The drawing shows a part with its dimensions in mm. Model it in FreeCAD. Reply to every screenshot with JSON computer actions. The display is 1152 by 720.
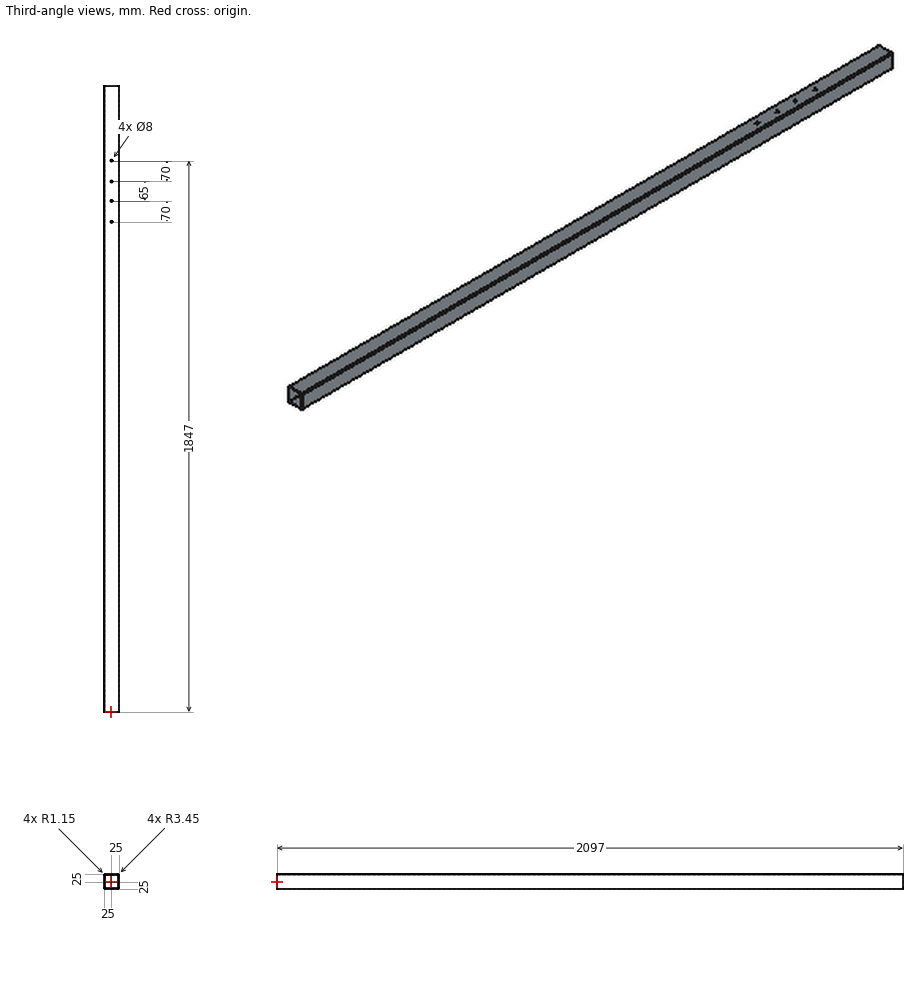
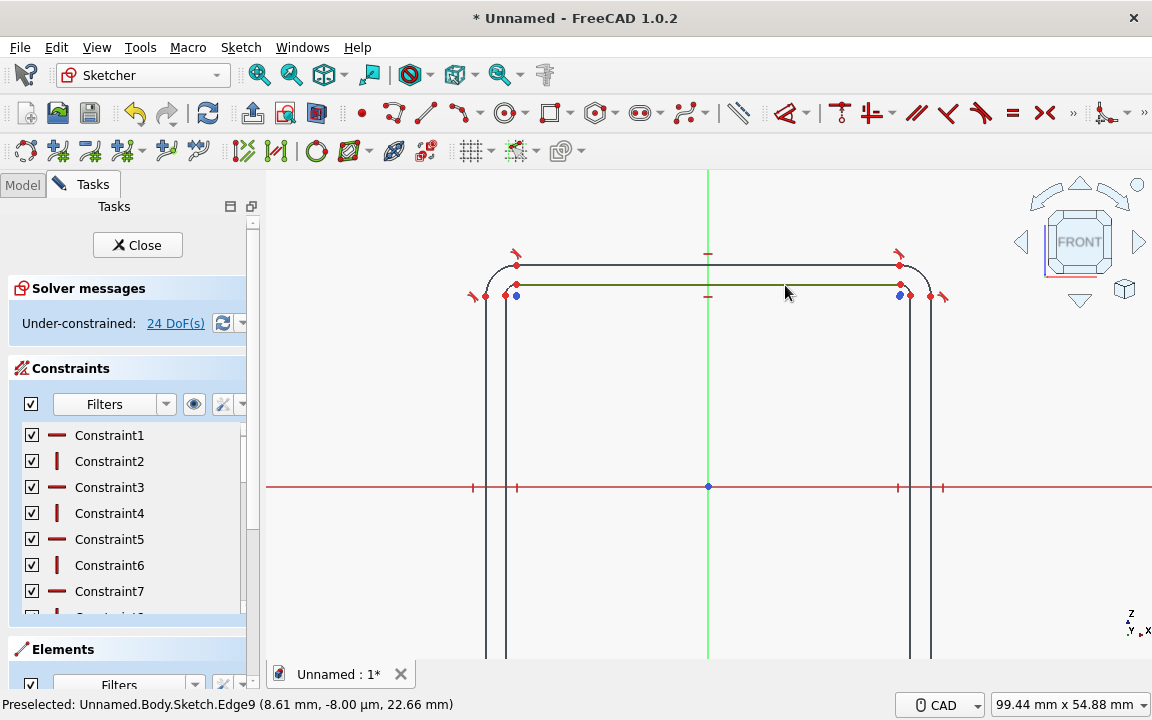
{"action": "scroll", "coordinate": [509, 288], "scroll_direction": "up", "scroll_amount": 3}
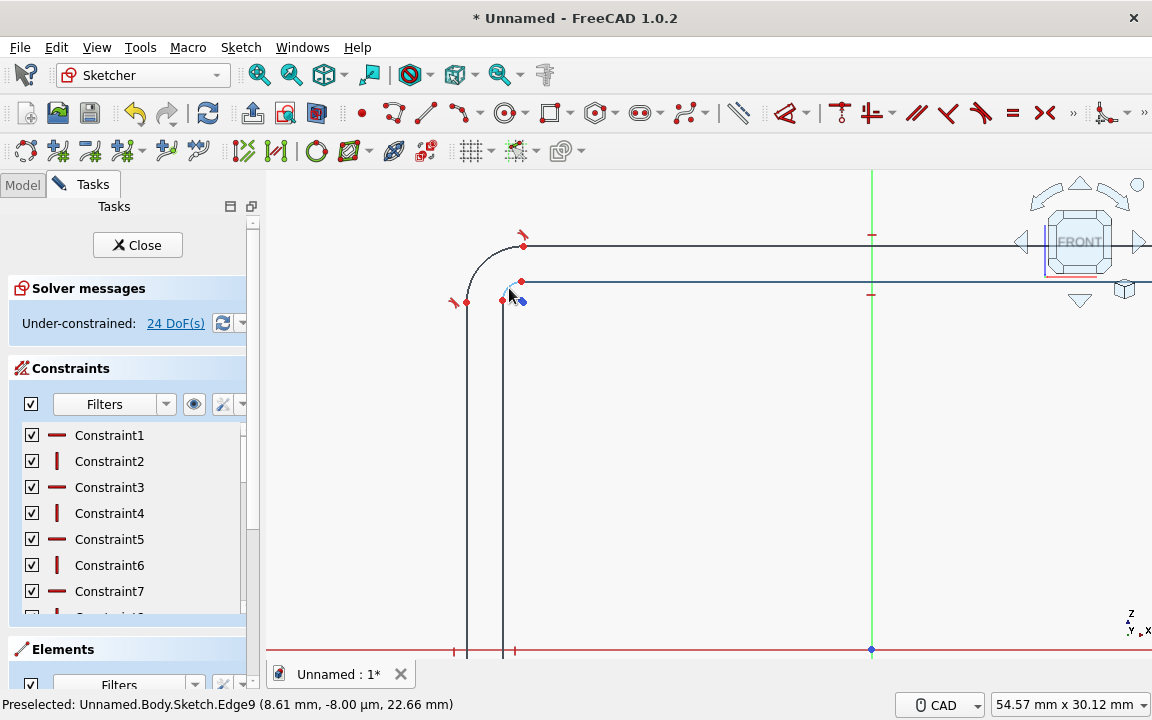
{"action": "left_click", "coordinate": [508, 287]}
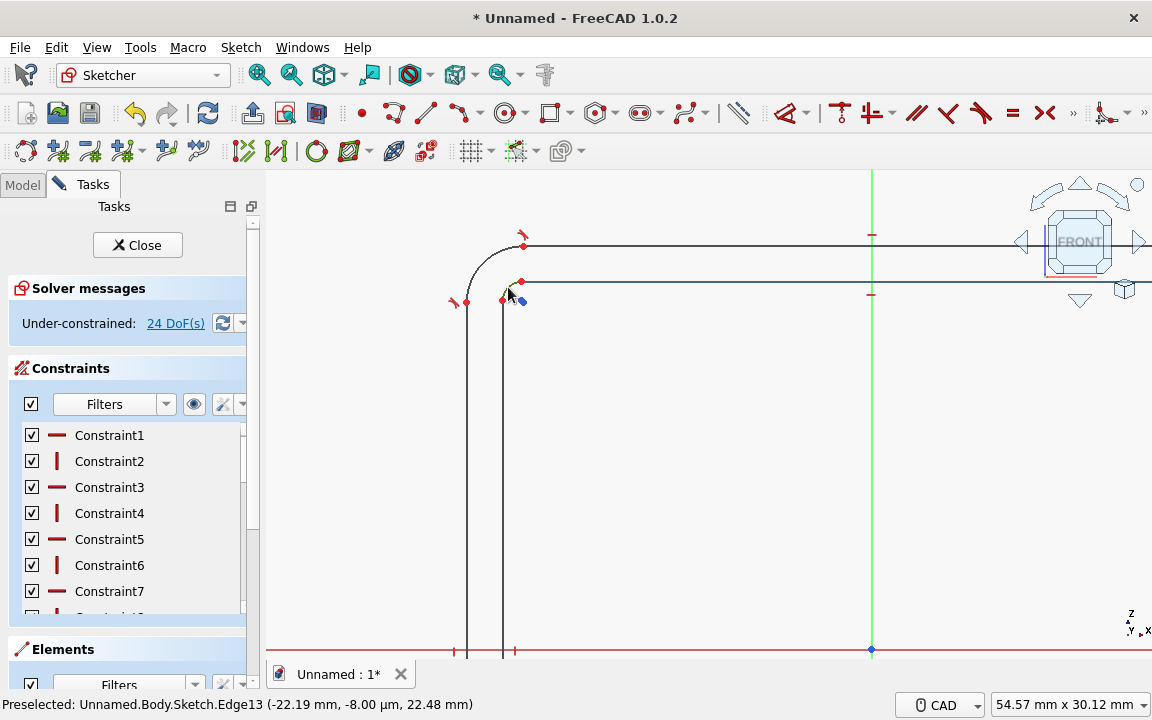
{"action": "left_click", "coordinate": [982, 114]}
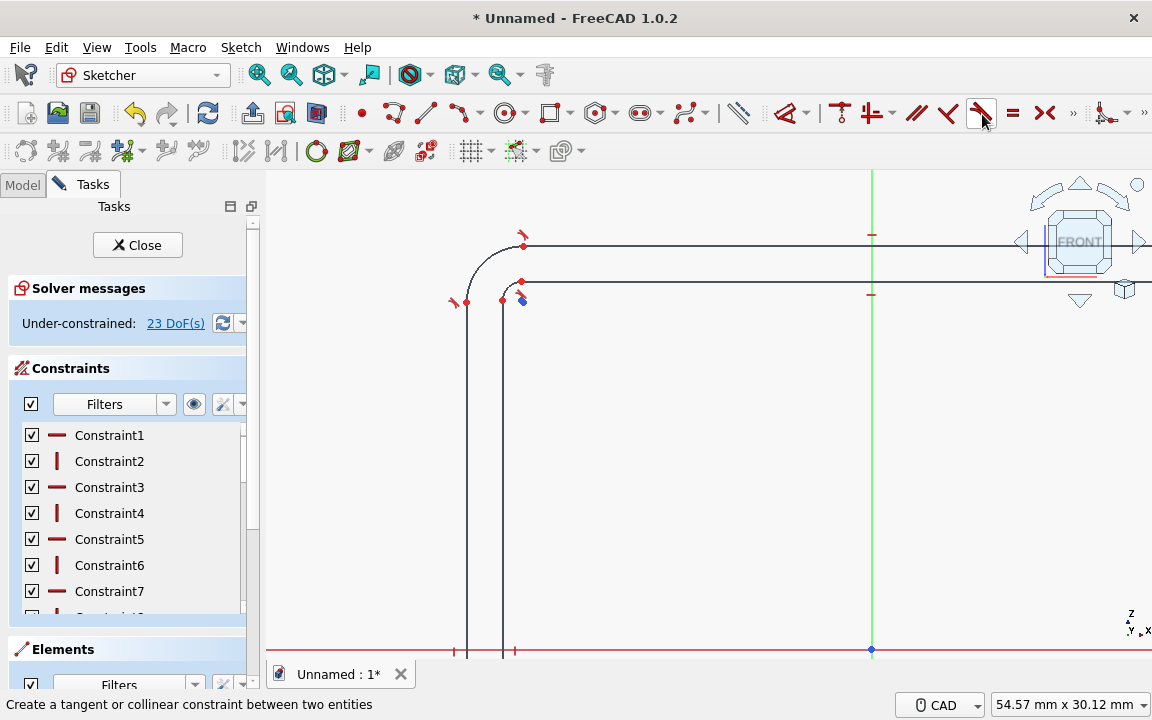
{"action": "left_click", "coordinate": [732, 282]}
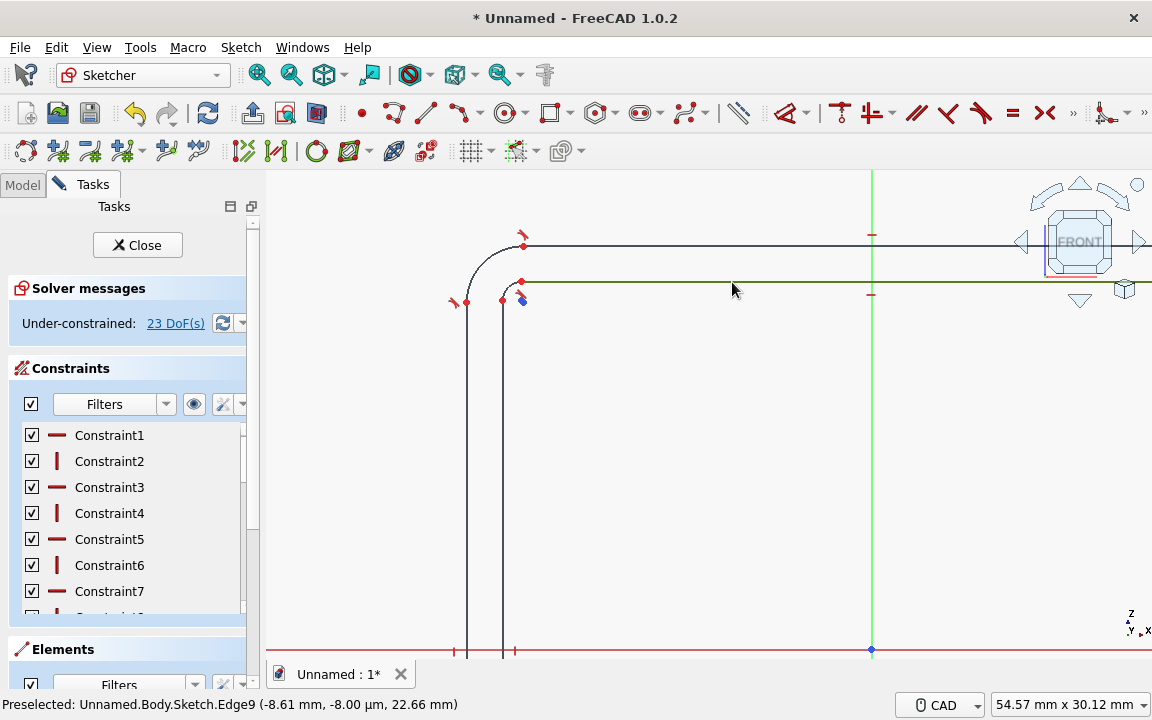
{"action": "scroll", "coordinate": [506, 278], "scroll_direction": "down", "scroll_amount": 5}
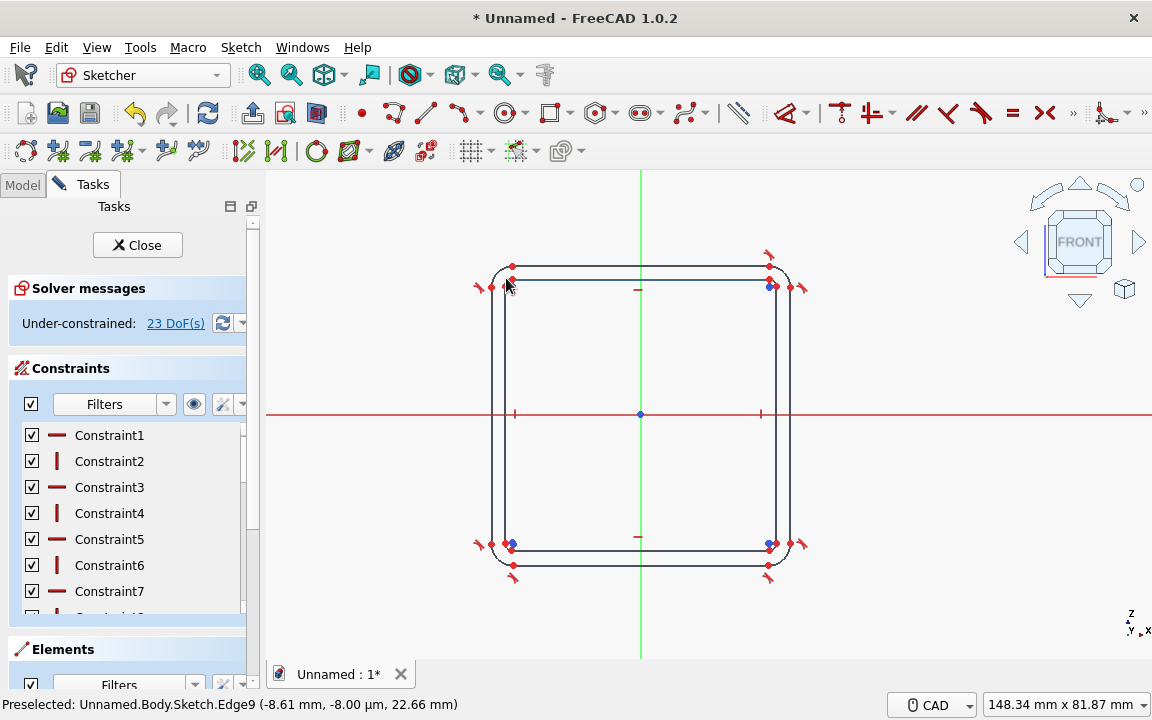
{"action": "scroll", "coordinate": [774, 282], "scroll_direction": "up", "scroll_amount": 5}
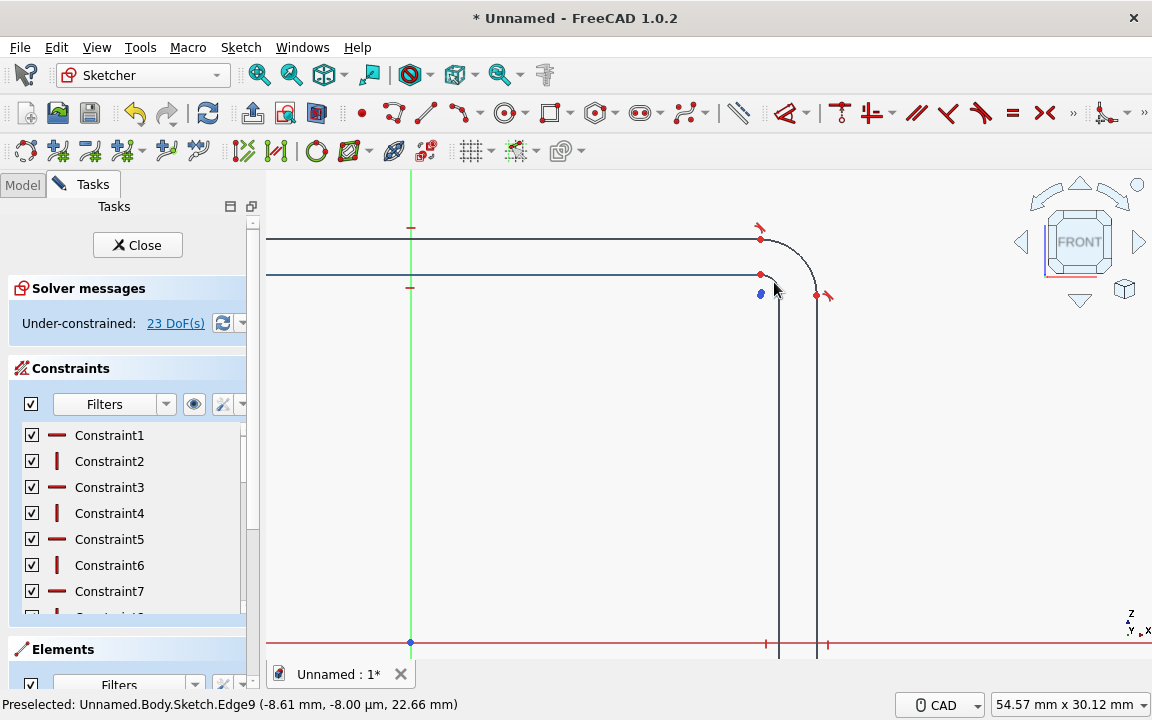
{"action": "left_click", "coordinate": [774, 281]}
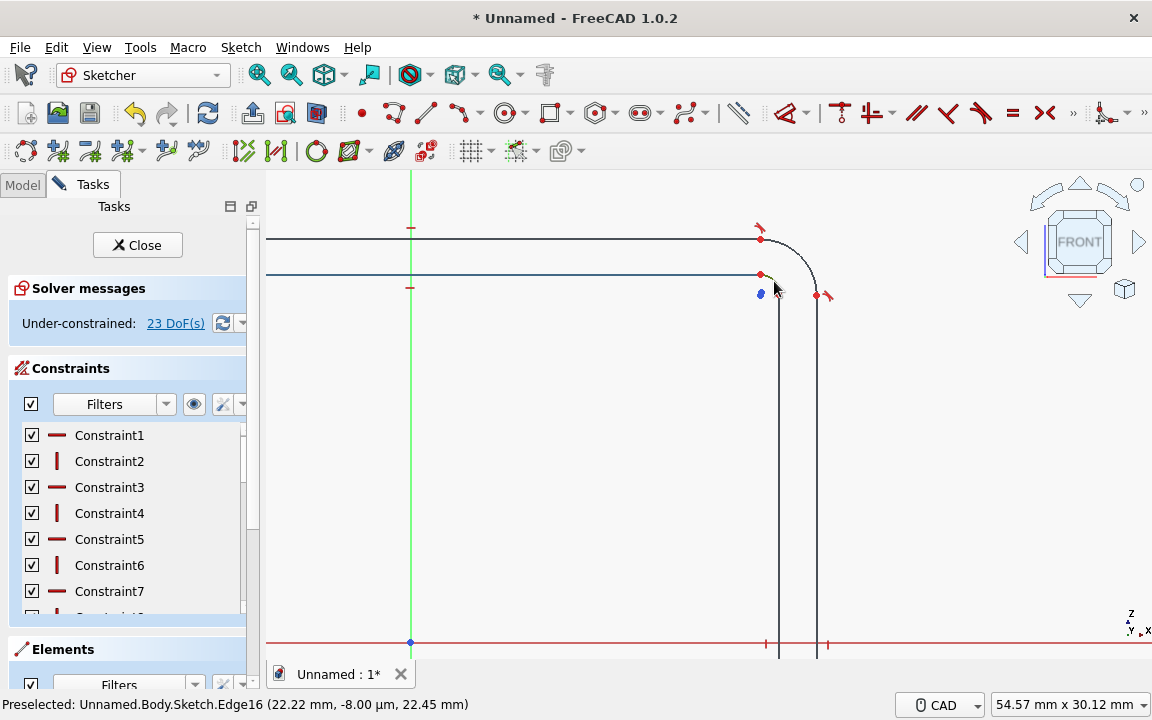
{"action": "left_click", "coordinate": [982, 114]}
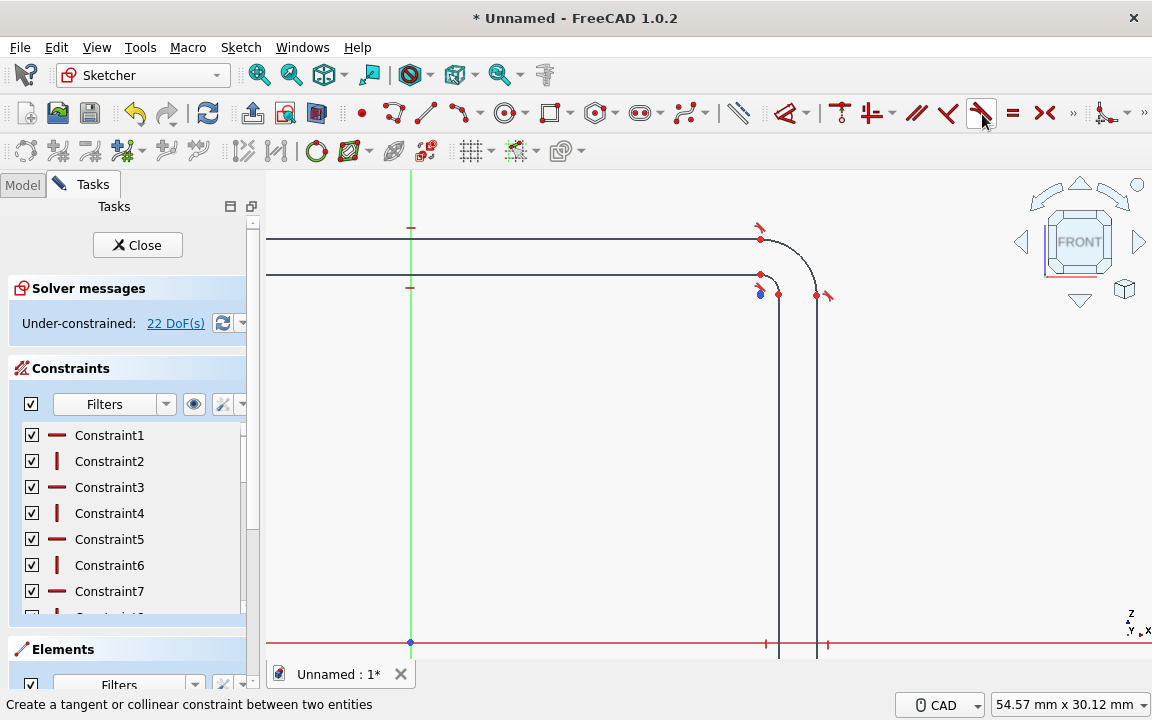
{"action": "scroll", "coordinate": [774, 282], "scroll_direction": "down", "scroll_amount": 5}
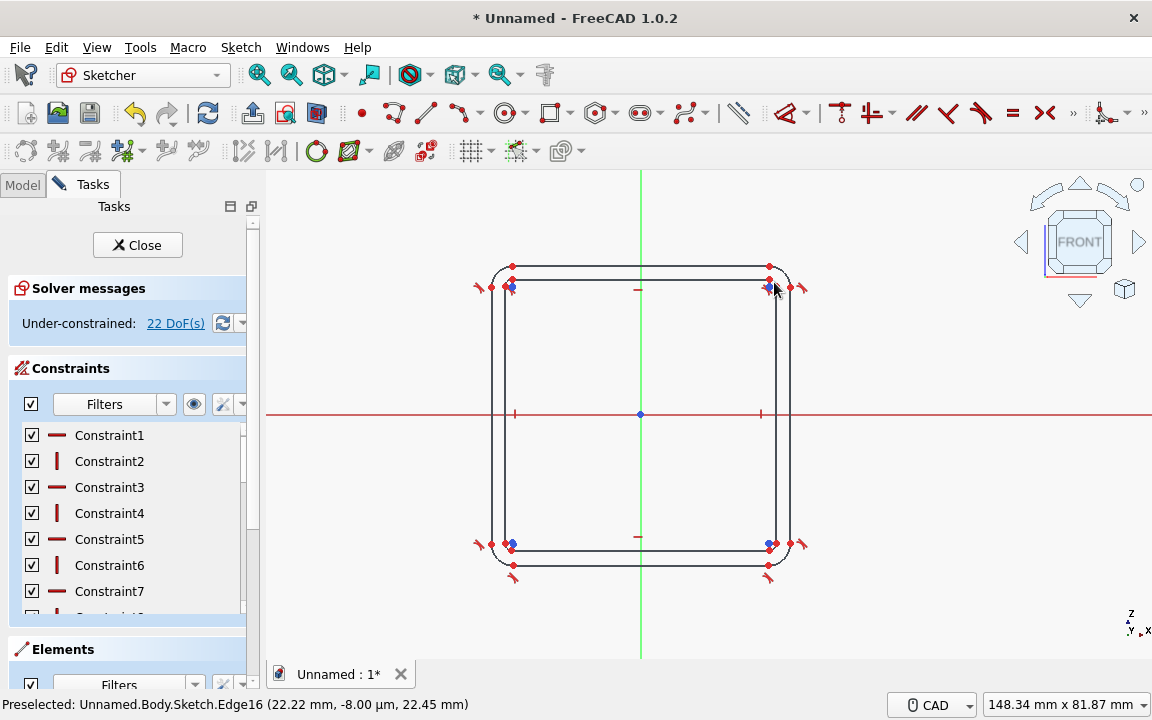
{"action": "left_click", "coordinate": [505, 364]}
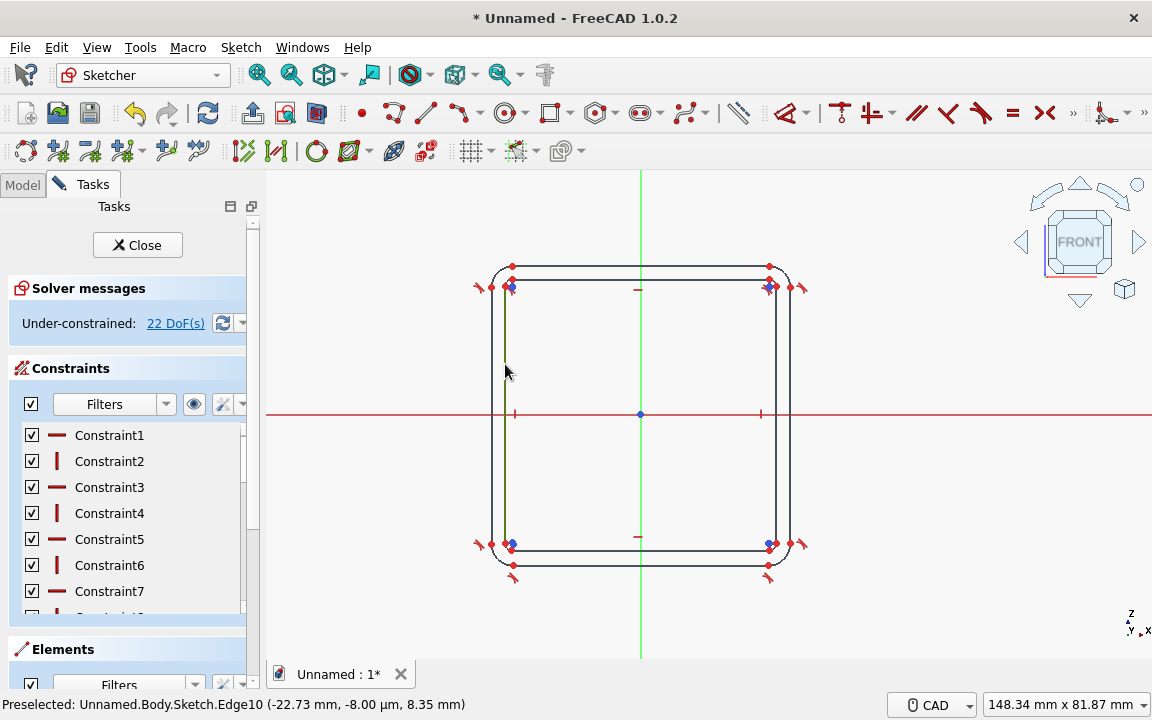
{"action": "scroll", "coordinate": [507, 282], "scroll_direction": "up", "scroll_amount": 5}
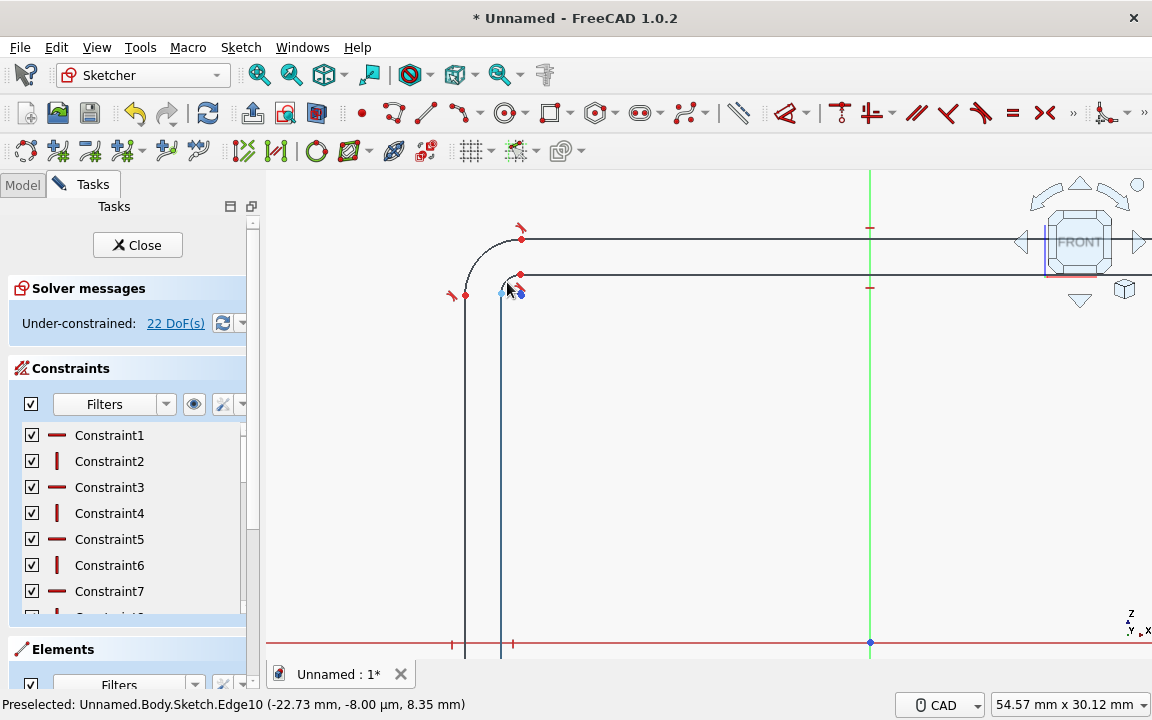
{"action": "left_click", "coordinate": [507, 281]}